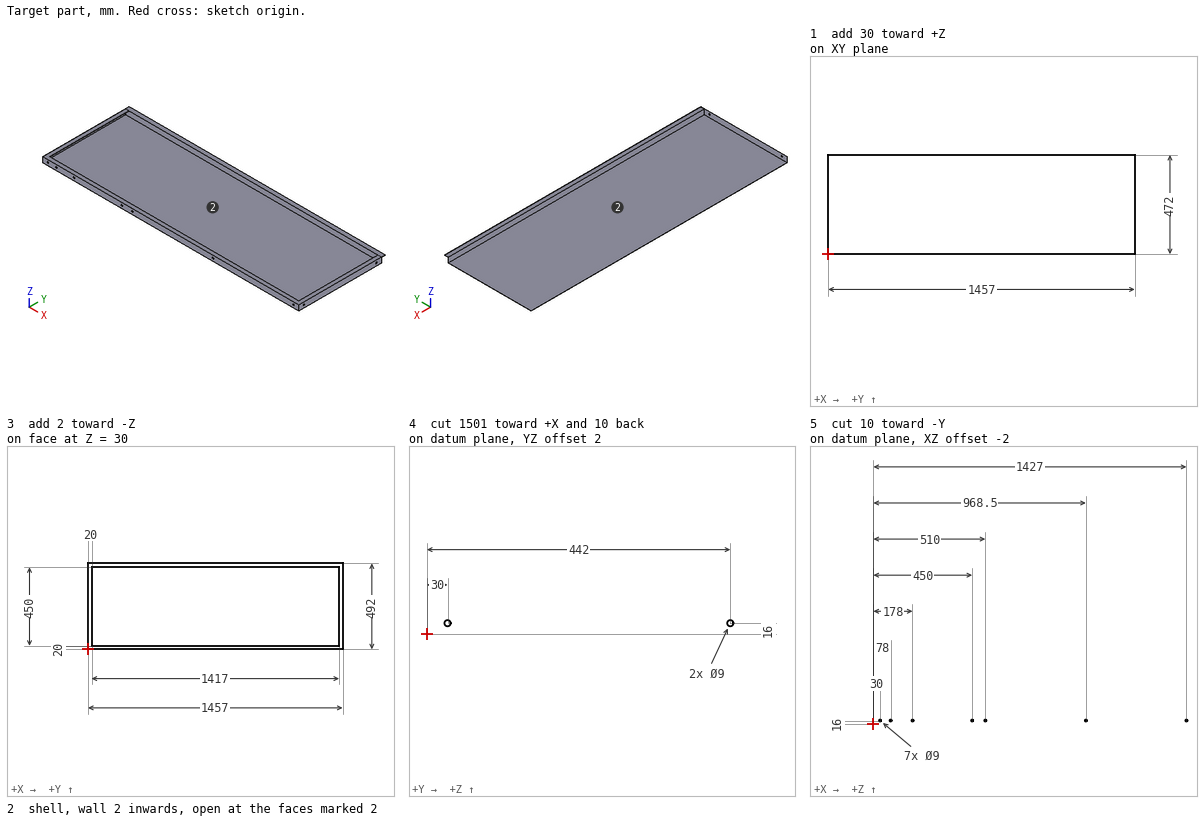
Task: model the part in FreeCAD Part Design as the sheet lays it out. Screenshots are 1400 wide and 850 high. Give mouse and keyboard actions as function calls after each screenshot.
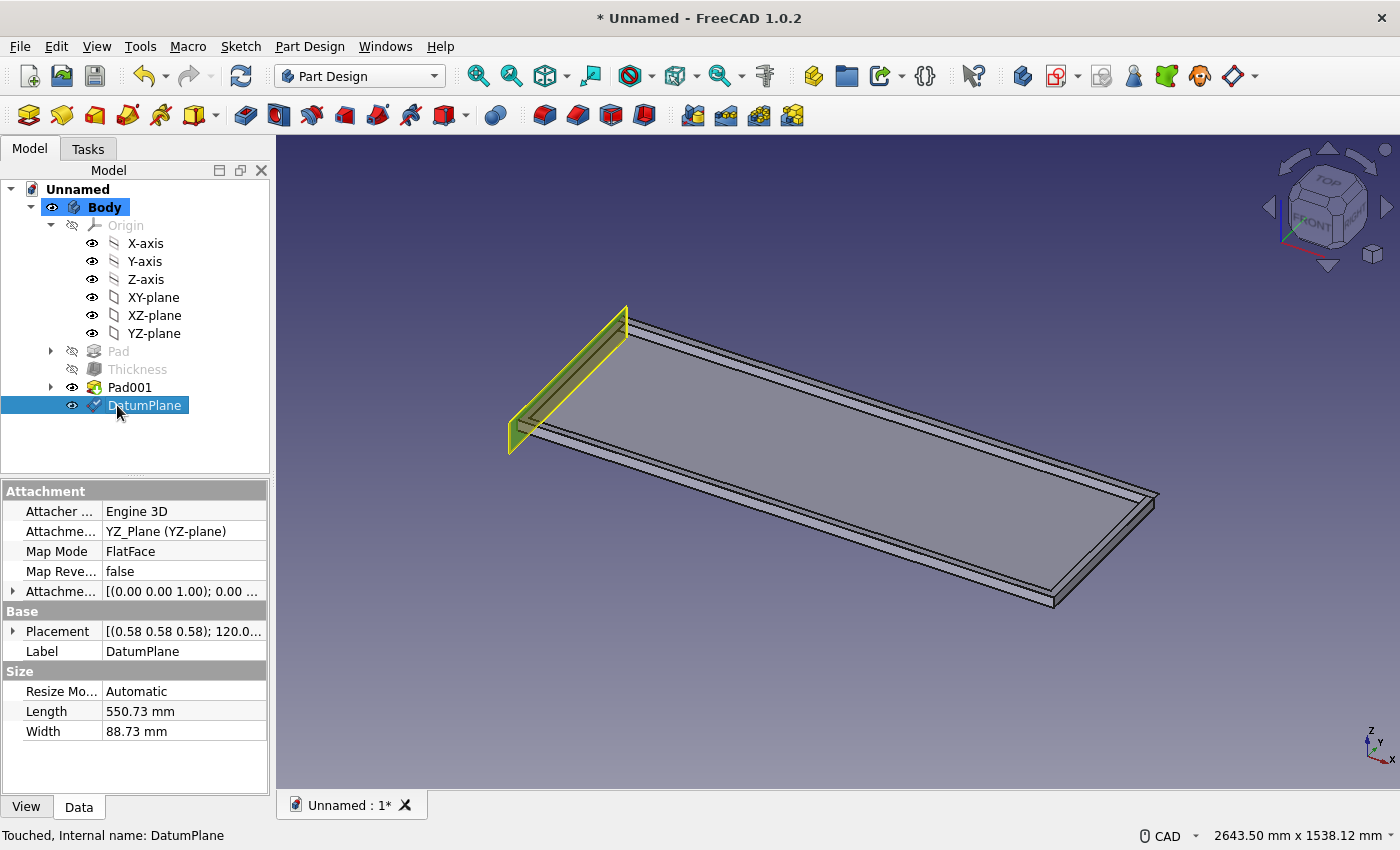
click(1056, 76)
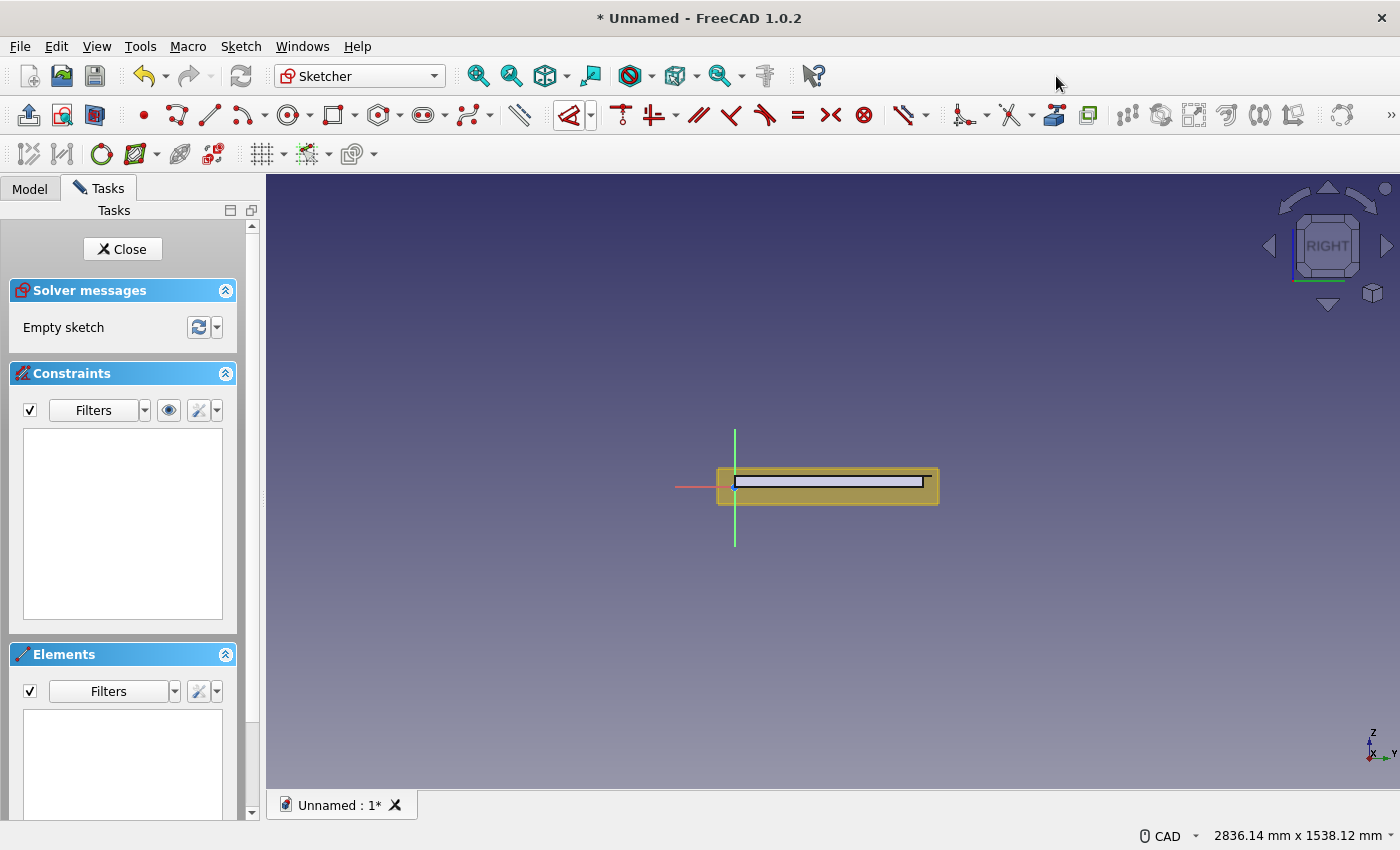
key(q)
key(s)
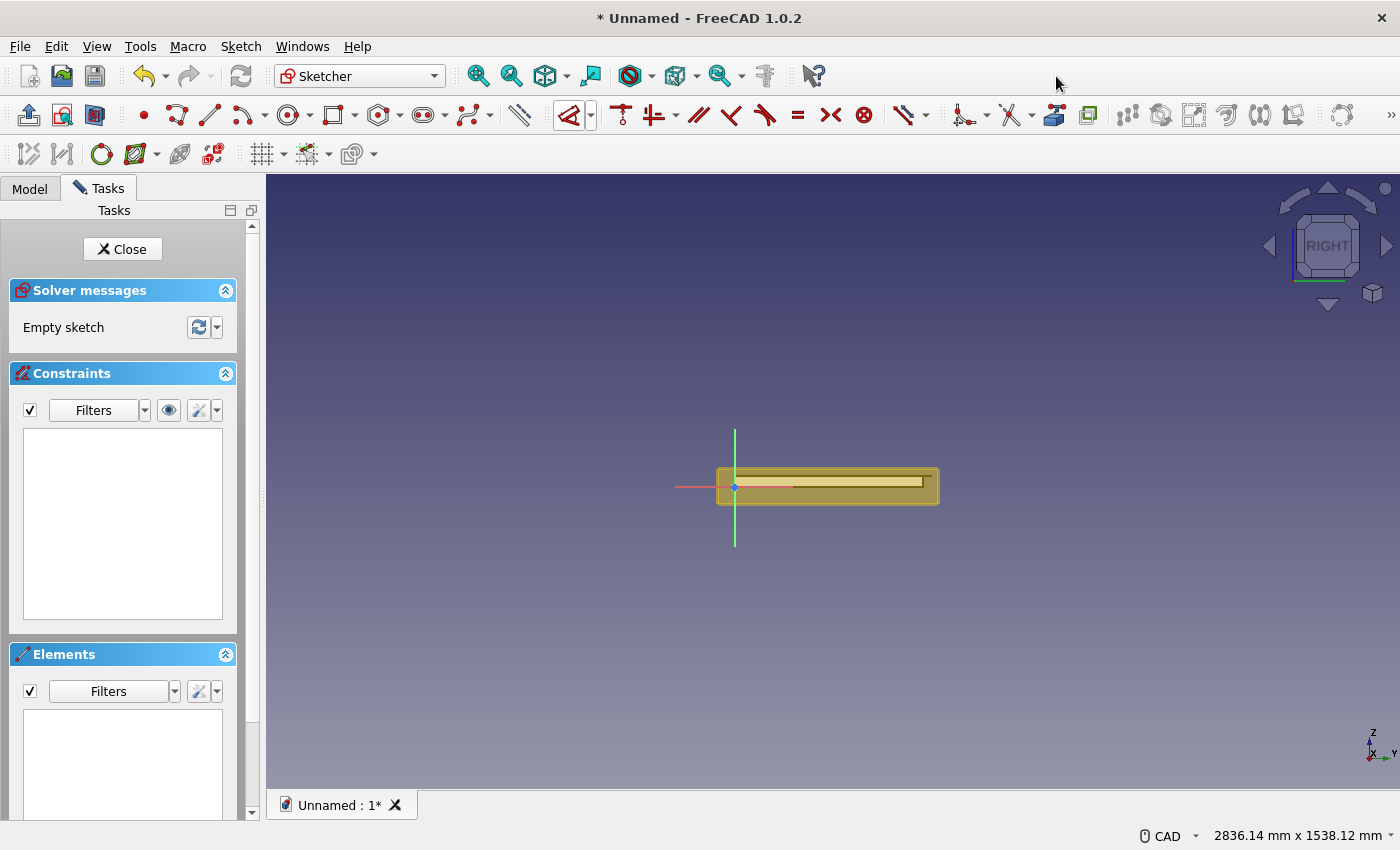
scroll(843, 484, up, 7)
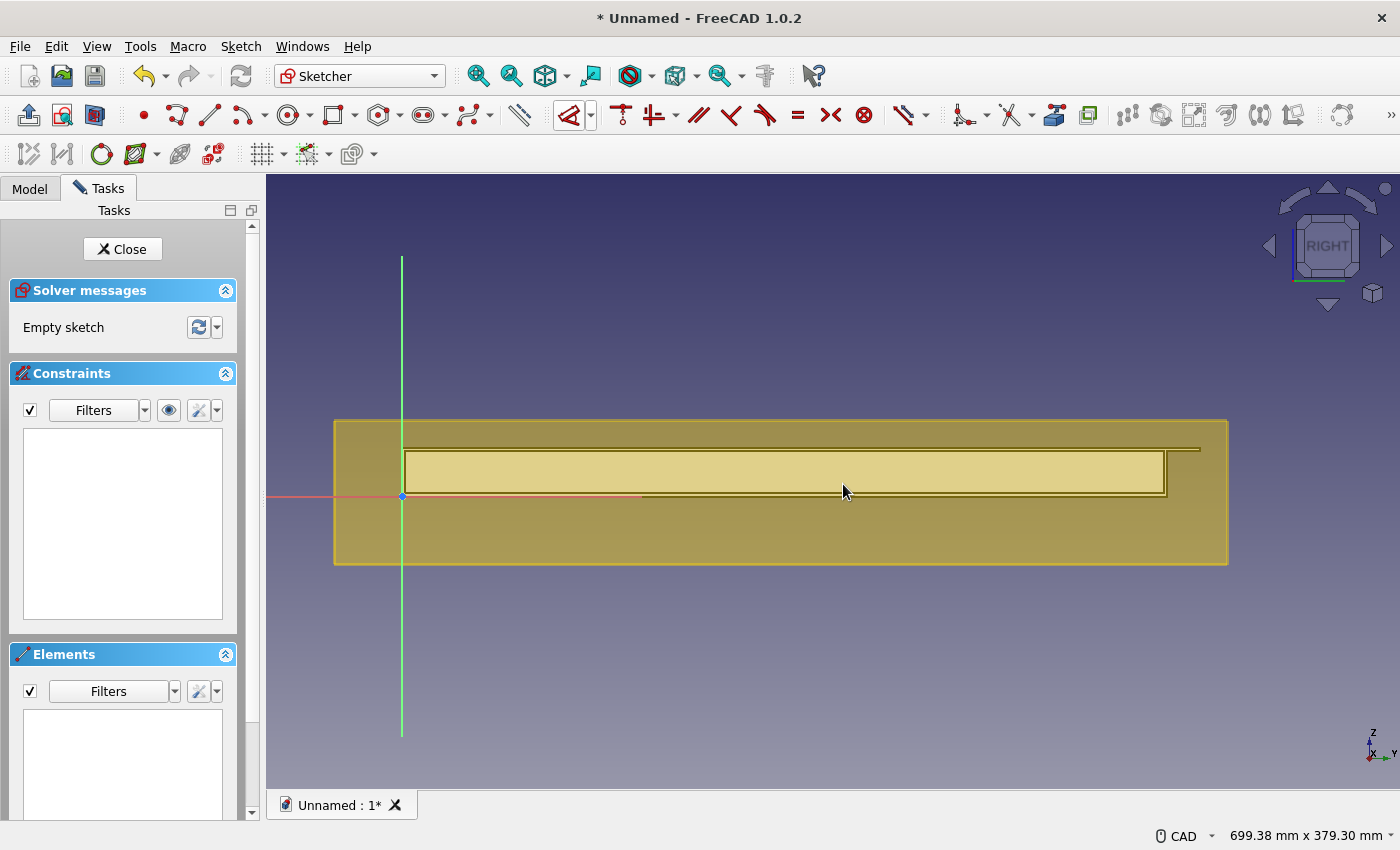
click(288, 116)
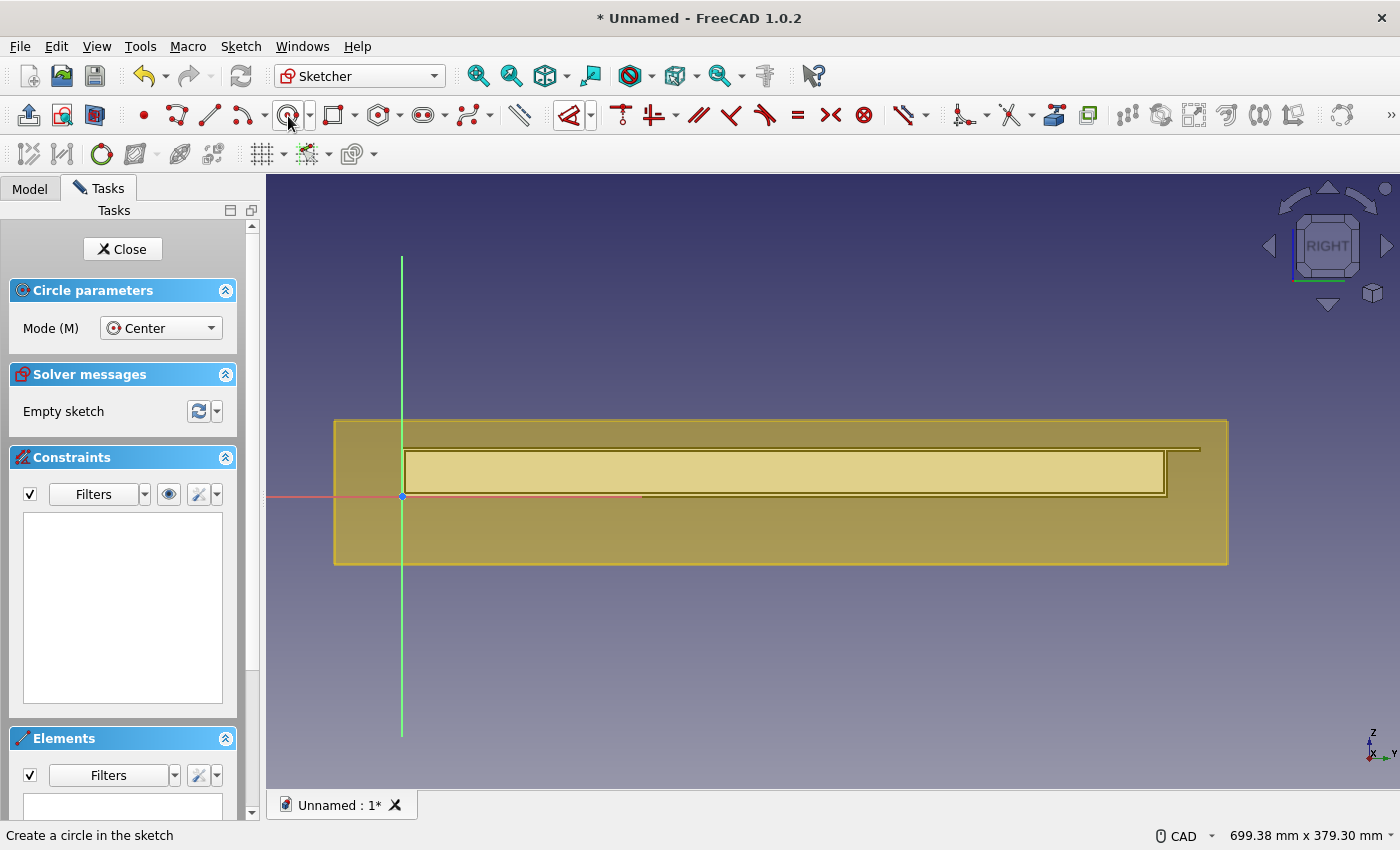
scroll(1119, 471, up, 6)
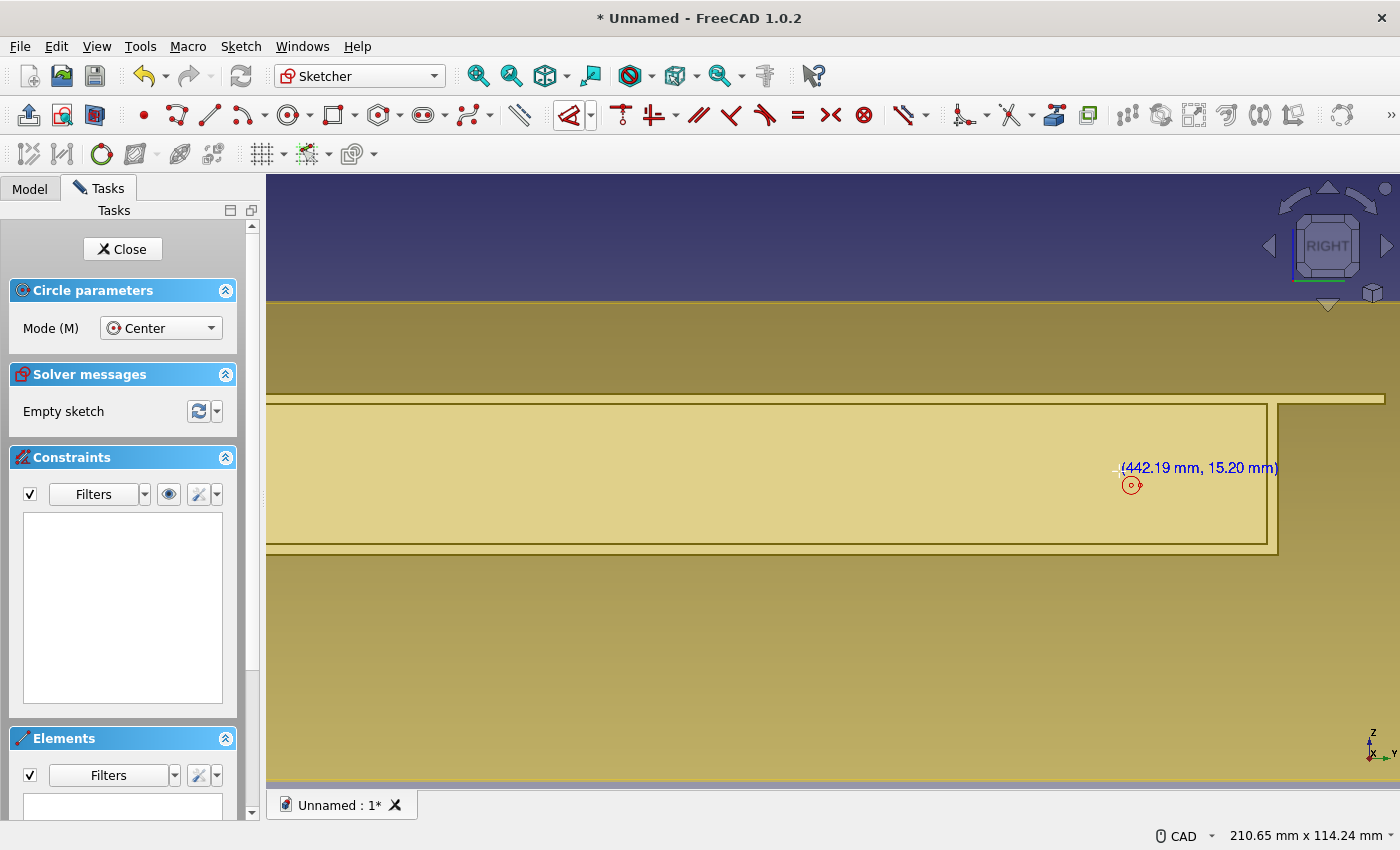
click(1116, 469)
move(1133, 452)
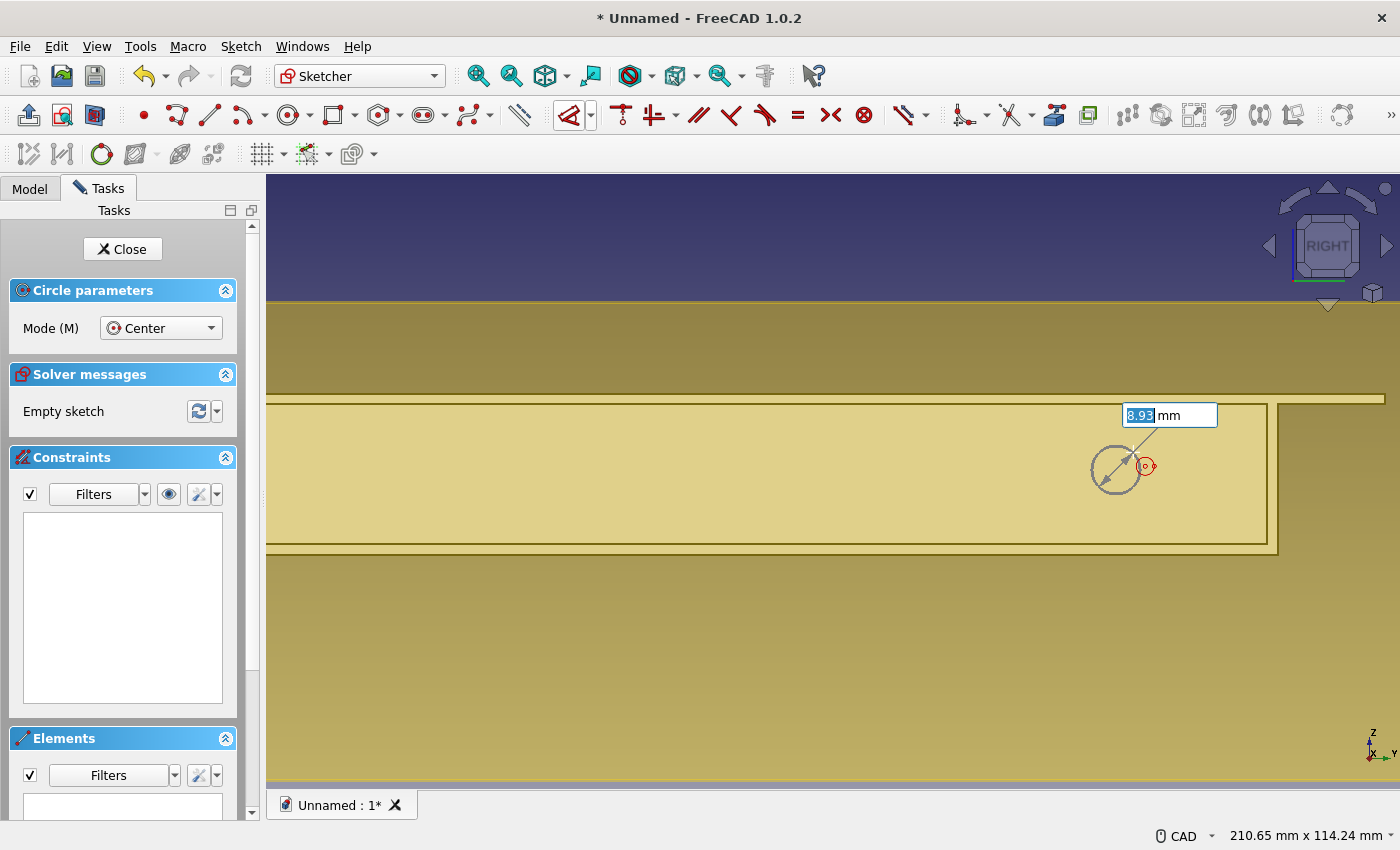
text(9)
key(Return)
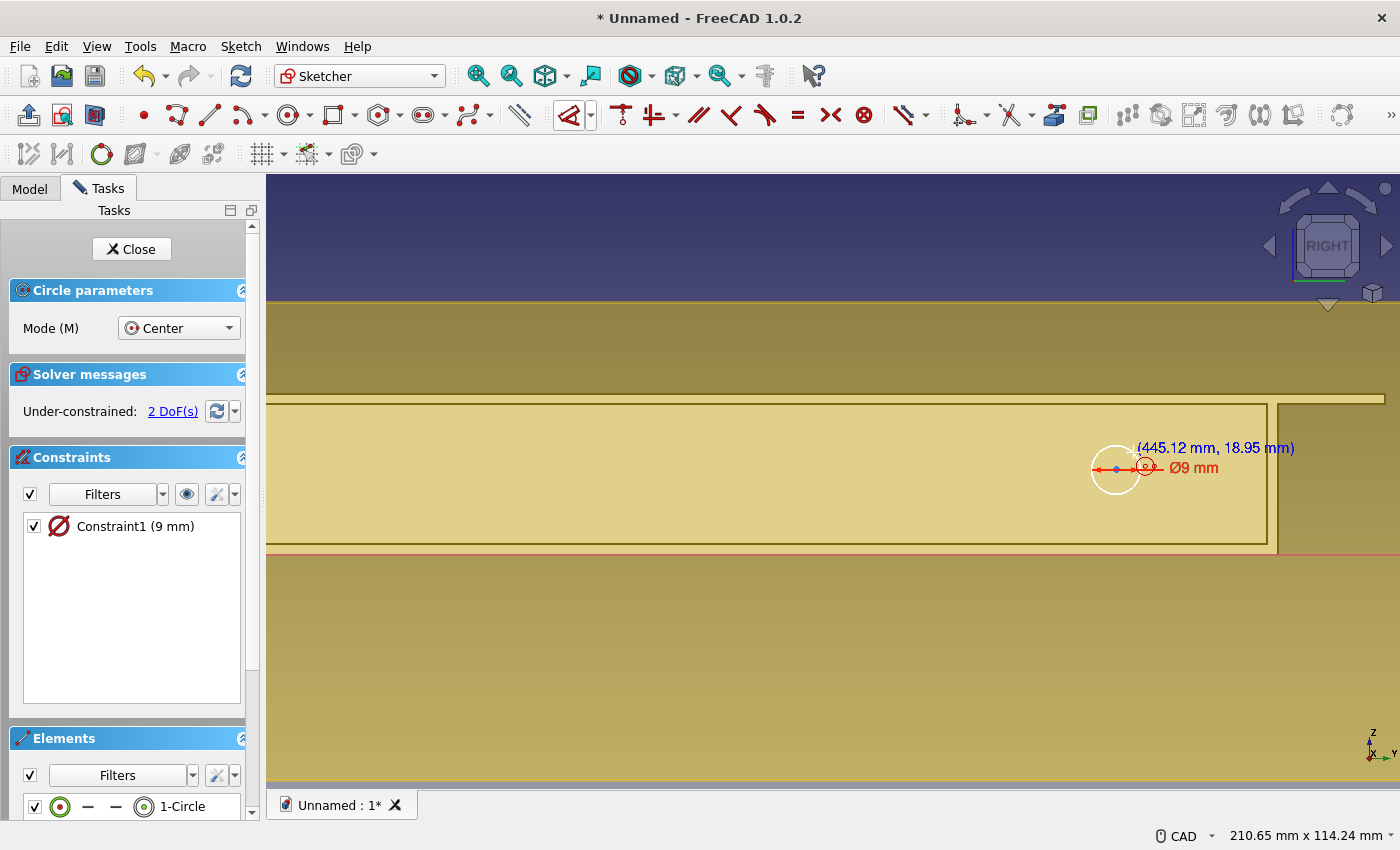
scroll(1120, 474, down, 6)